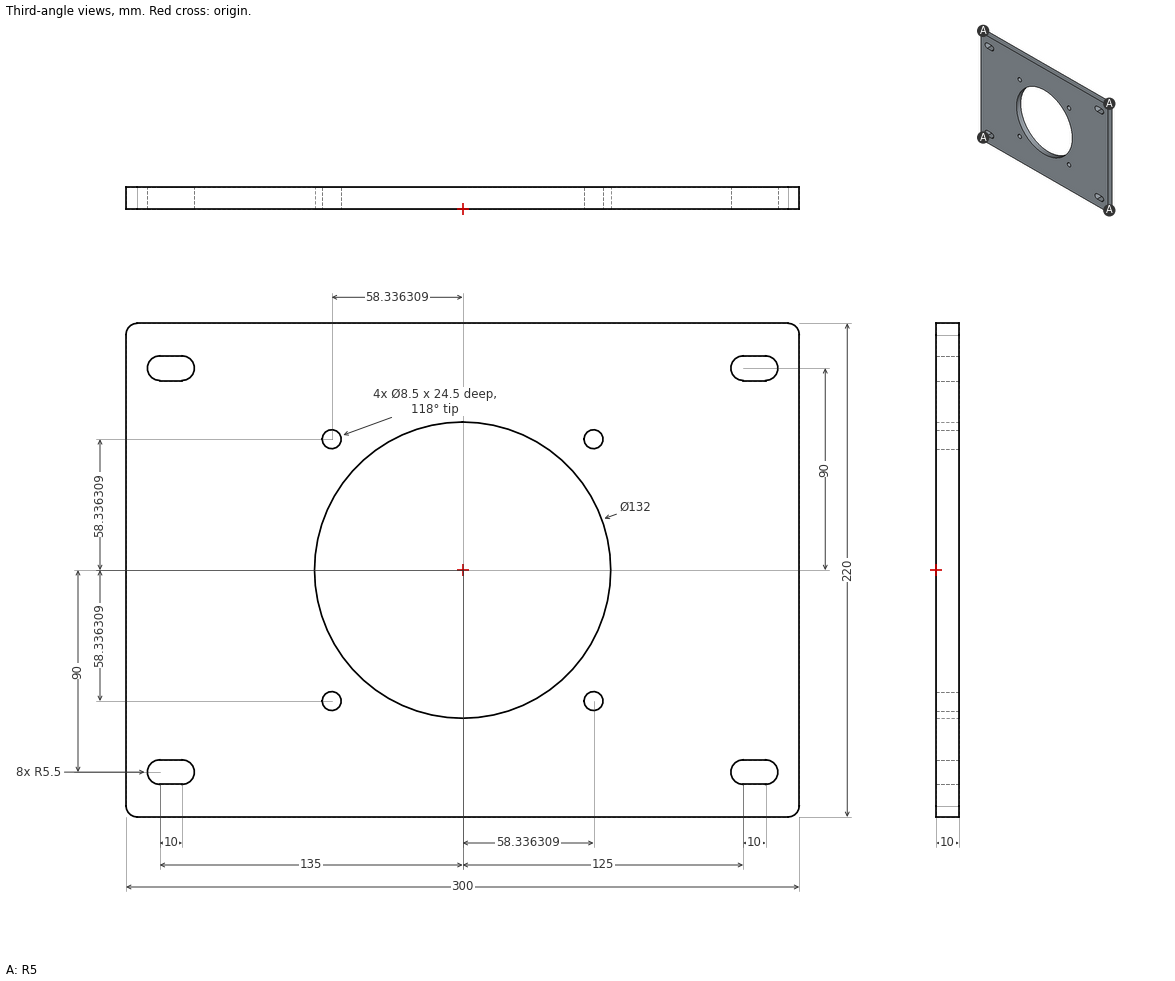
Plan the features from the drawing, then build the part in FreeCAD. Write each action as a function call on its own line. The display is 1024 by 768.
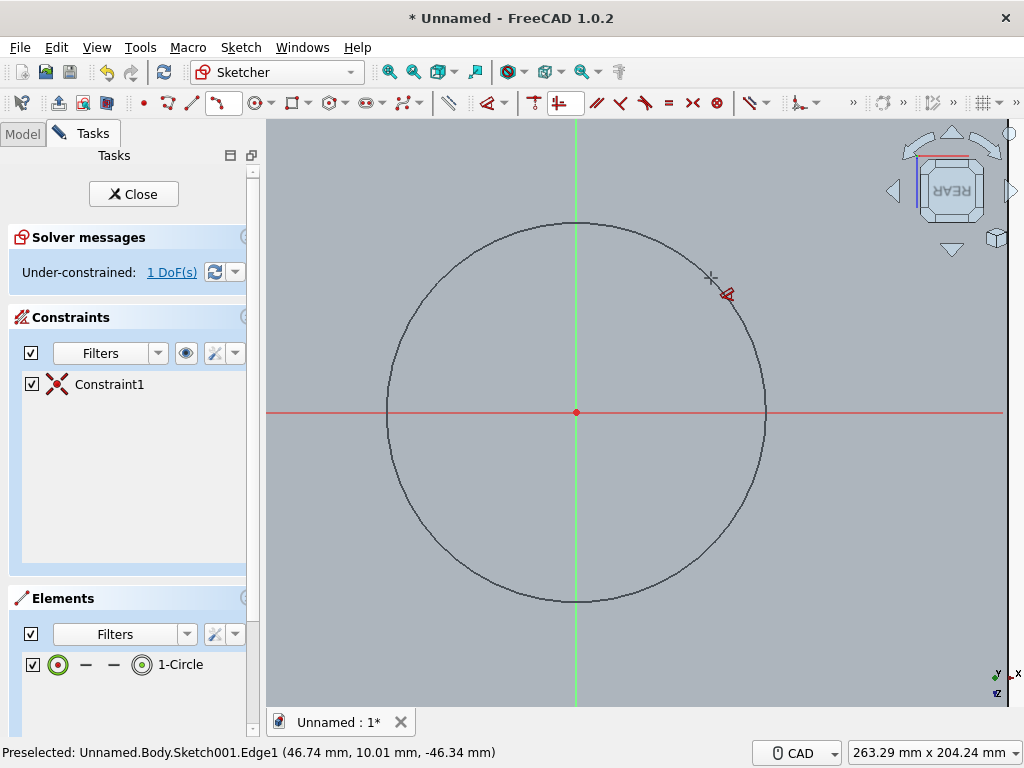
click(710, 278)
click(733, 255)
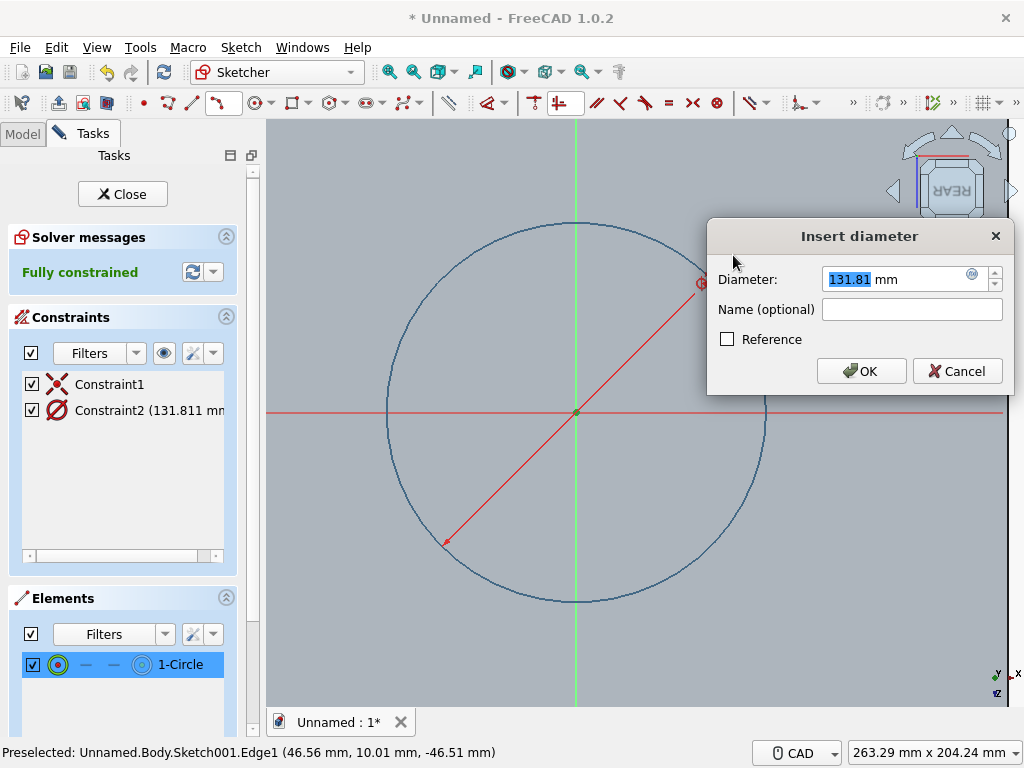
text(132)
key(Return)
key(Escape)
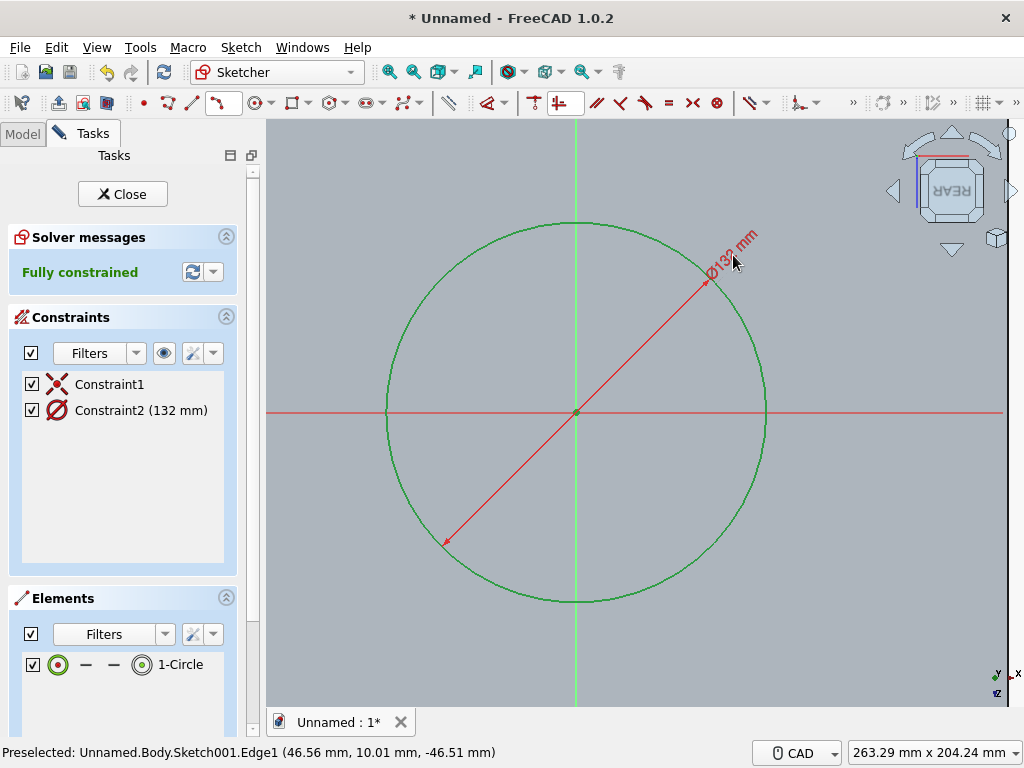
click(123, 194)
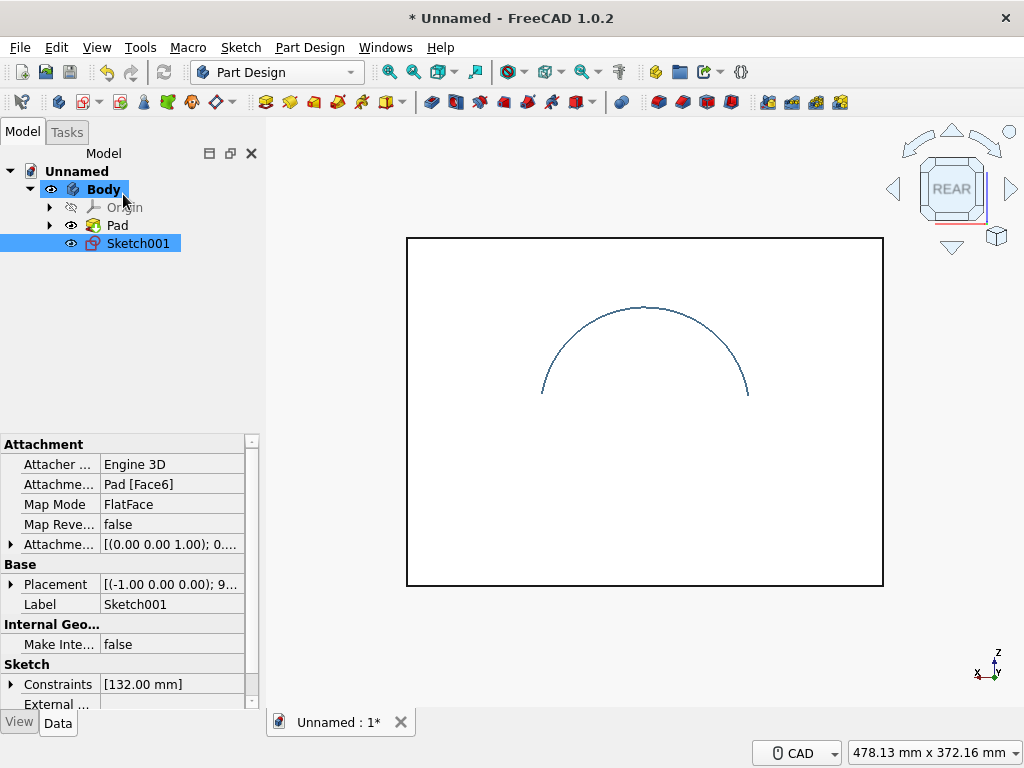
click(432, 102)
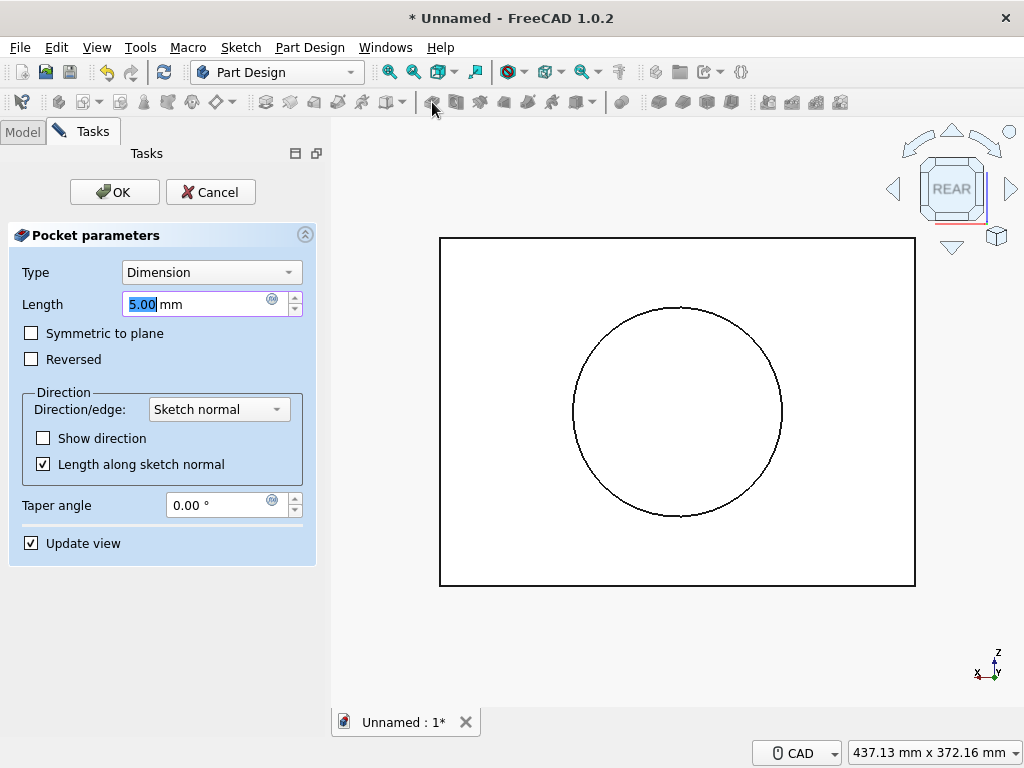
click(212, 272)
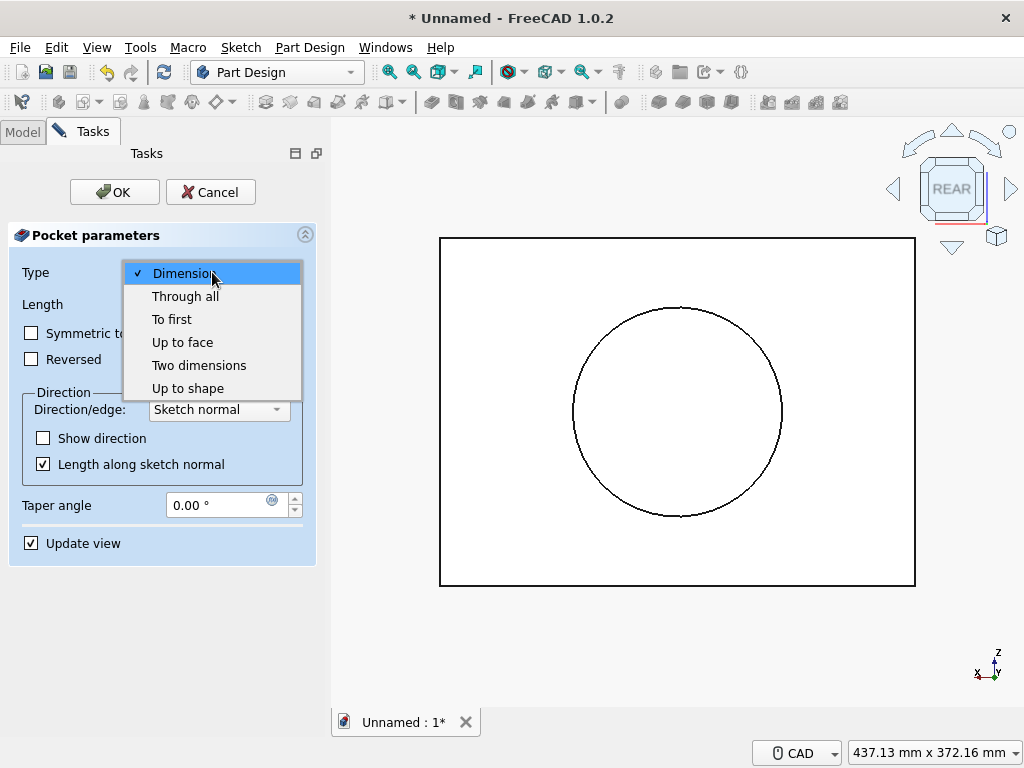
click(212, 296)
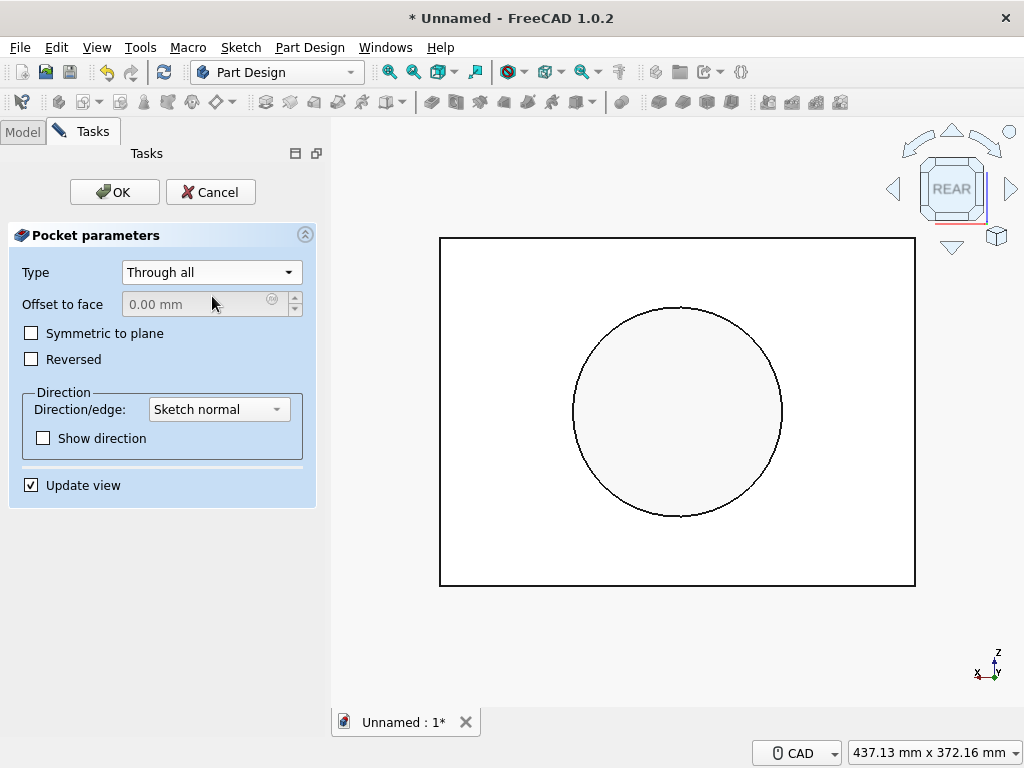
click(115, 192)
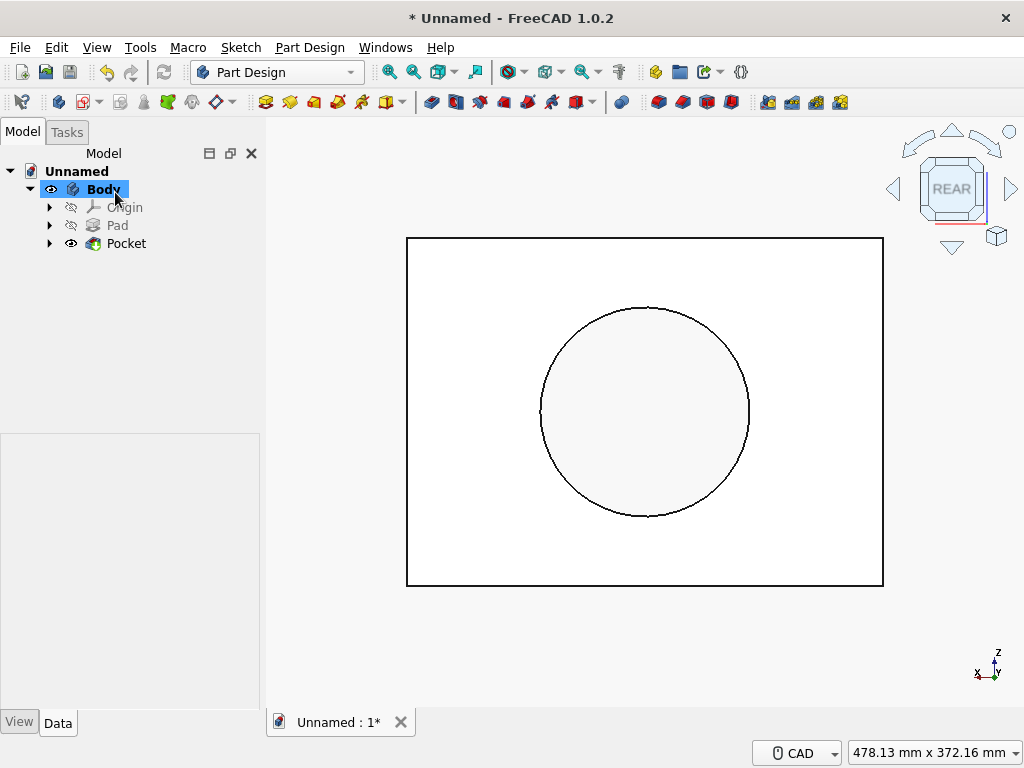
click(509, 311)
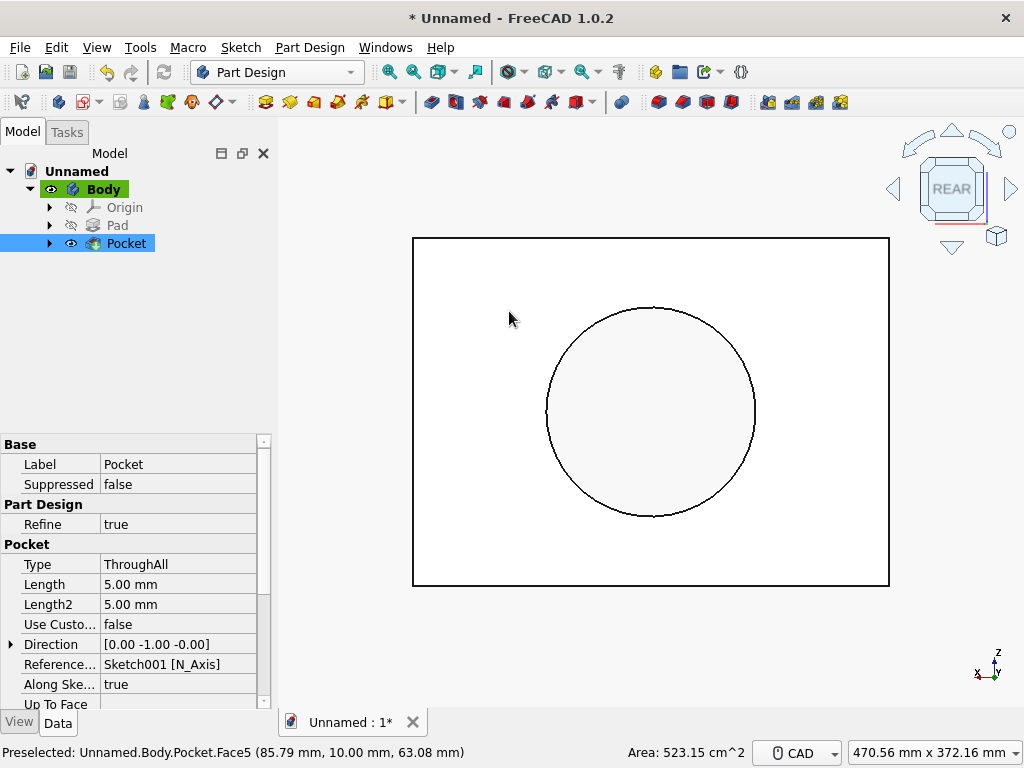
click(84, 102)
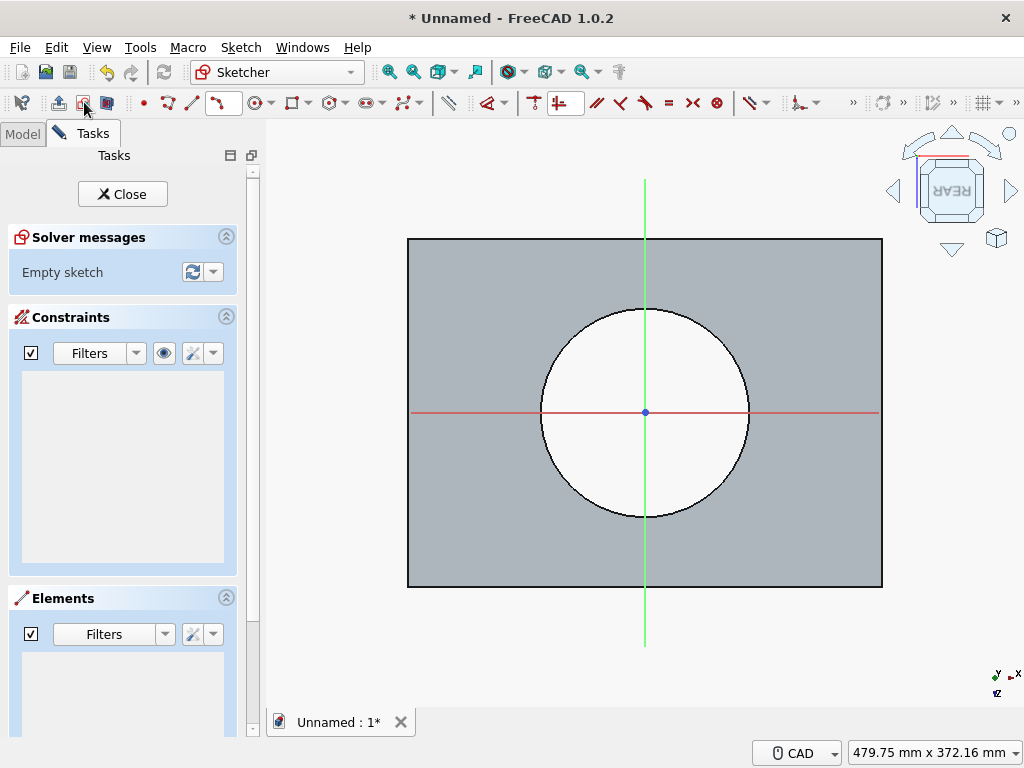
scroll(728, 413, up, 3)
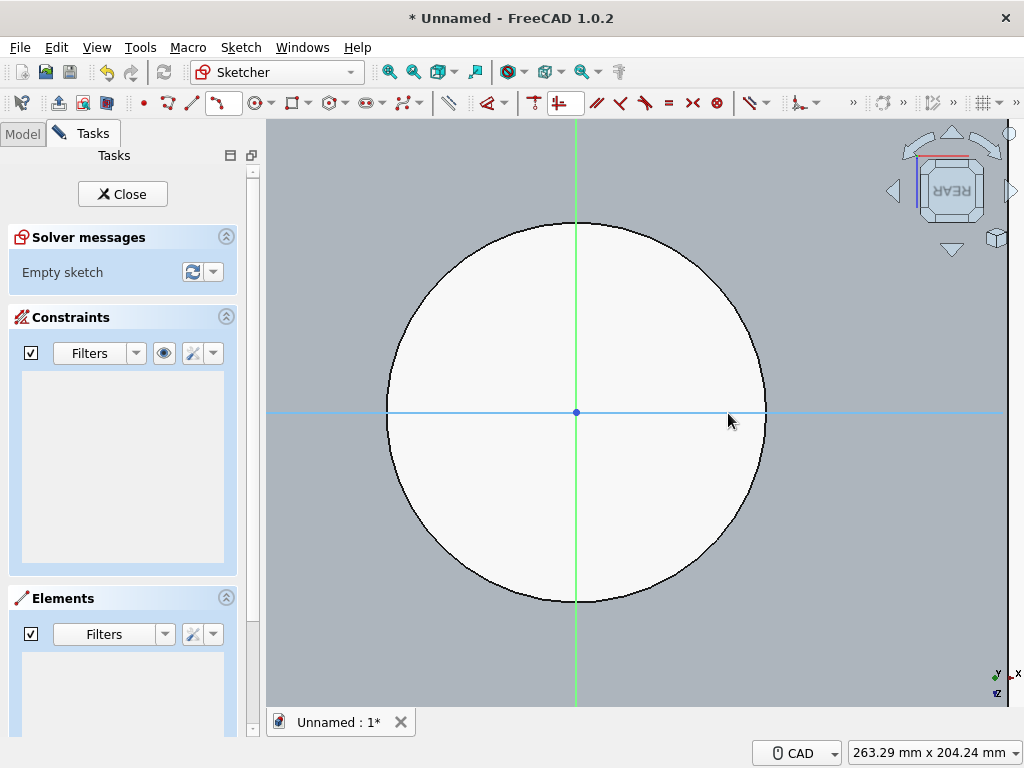
key(g)
key(c)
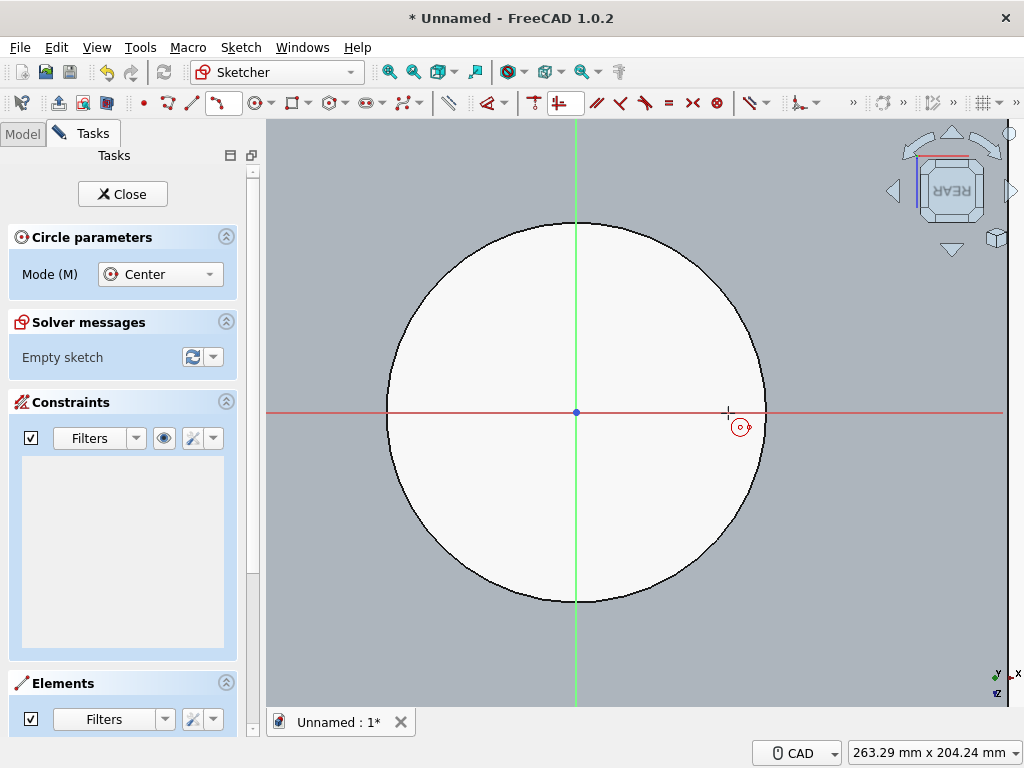
scroll(408, 581, up, 4)